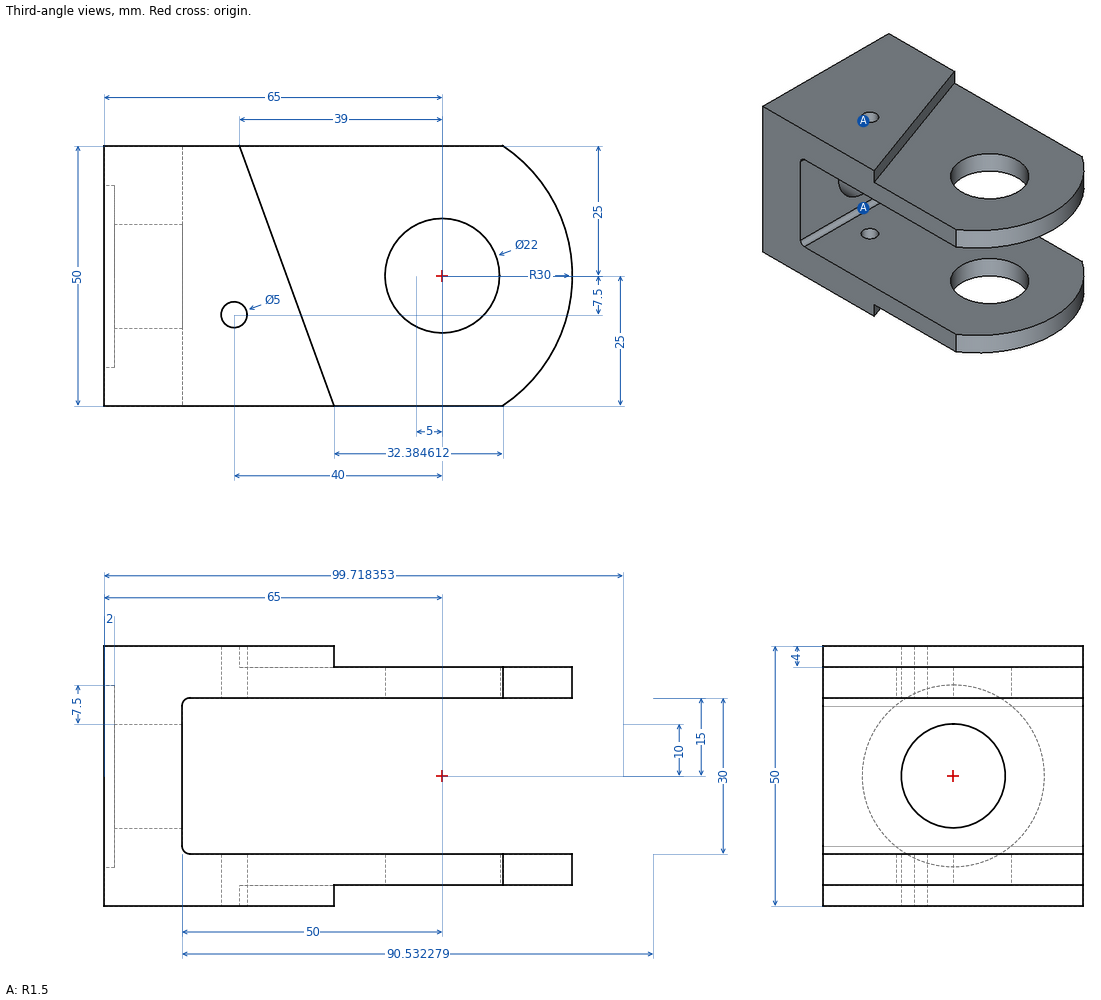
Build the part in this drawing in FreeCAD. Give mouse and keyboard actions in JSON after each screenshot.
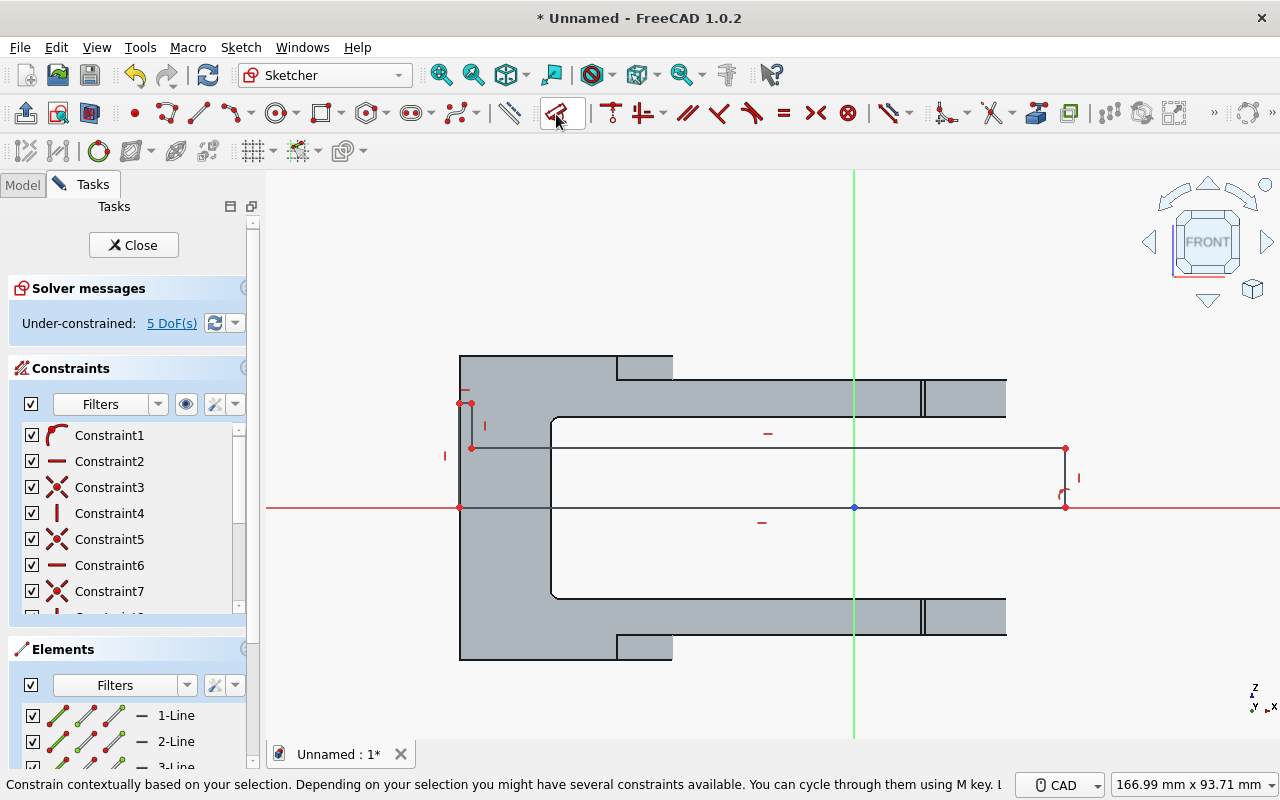
{"action": "scroll", "coordinate": [465, 403], "scroll_direction": "up", "scroll_amount": 6}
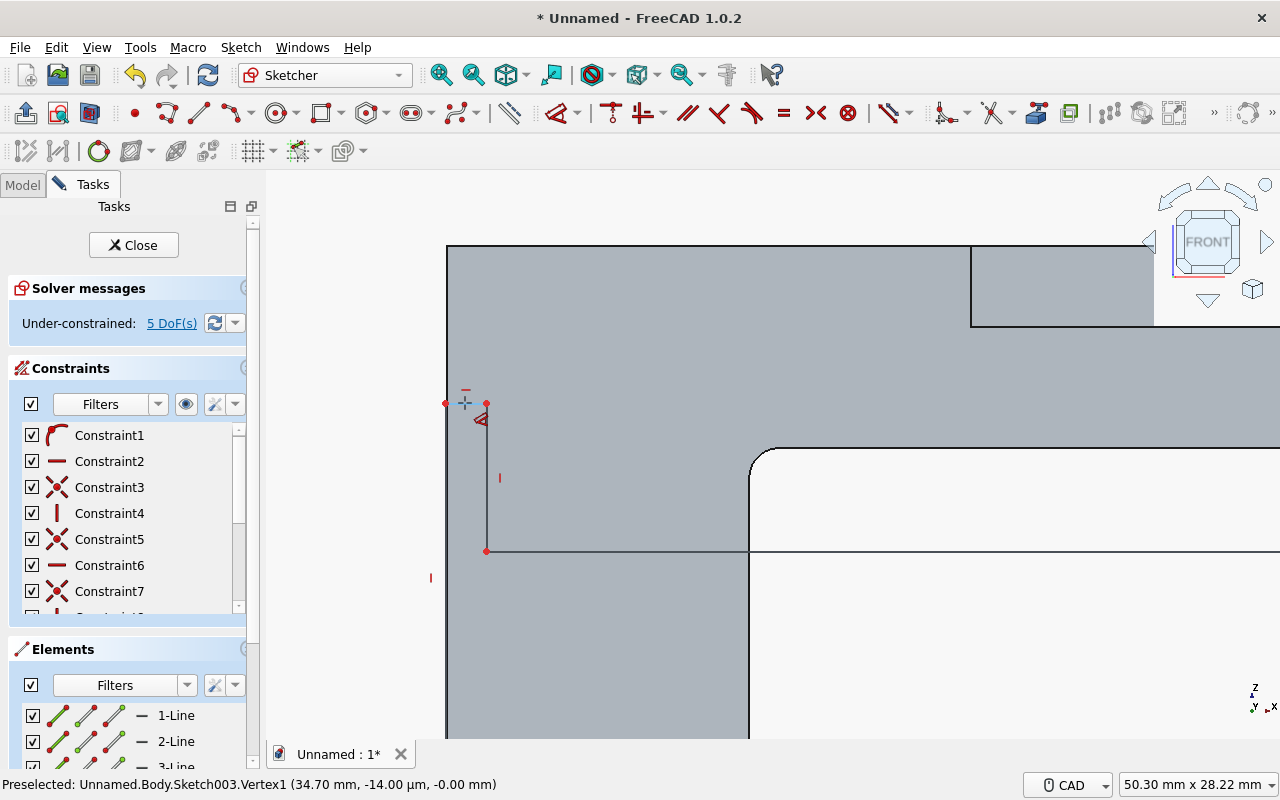
{"action": "left_click", "coordinate": [466, 404]}
{"action": "left_click", "coordinate": [466, 370]}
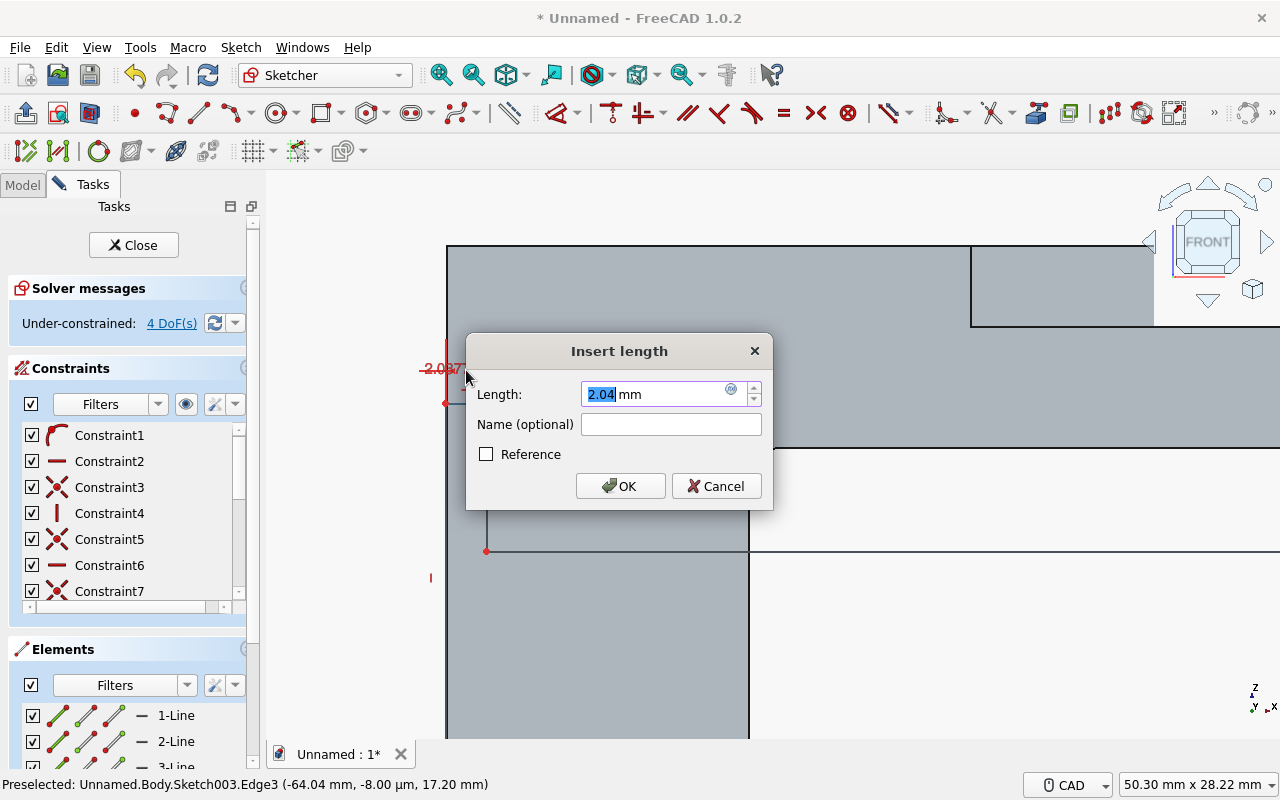
{"action": "type", "text": "2"}
{"action": "key", "text": "Return"}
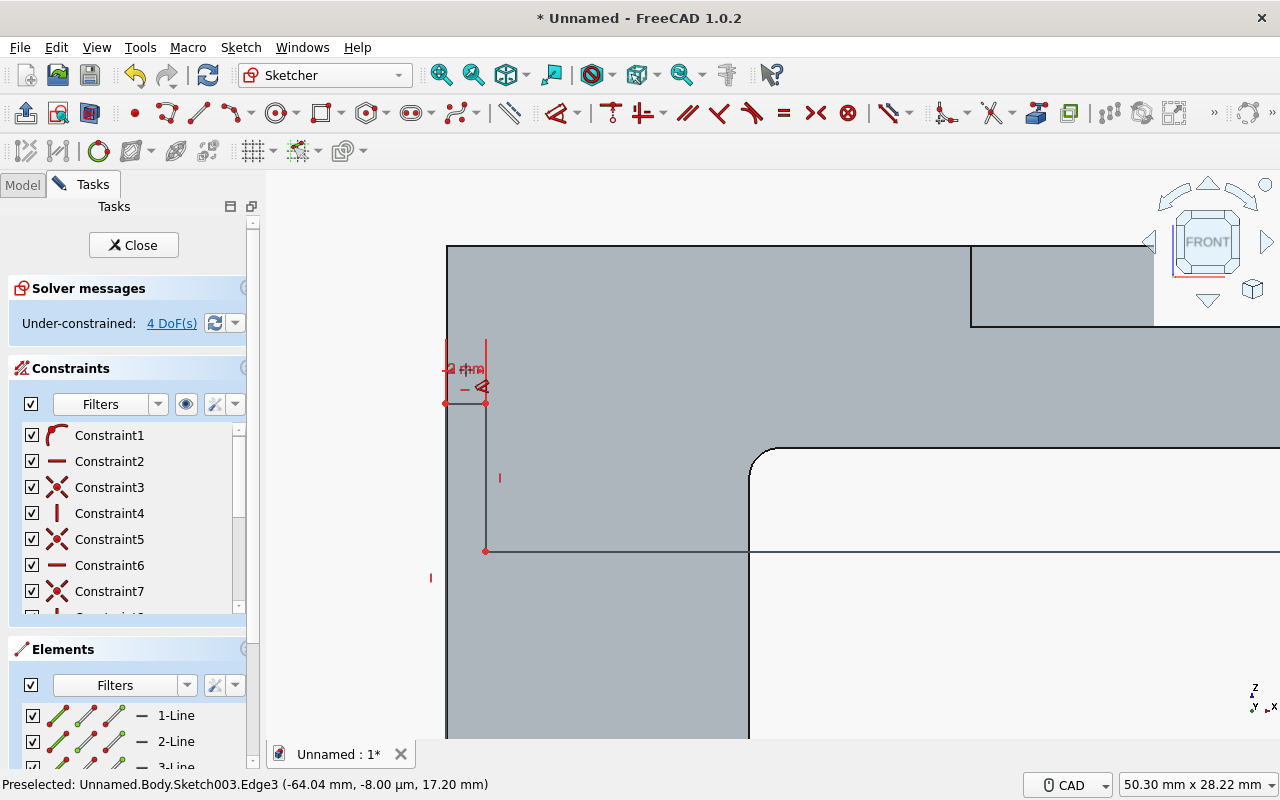
{"action": "scroll", "coordinate": [382, 403], "scroll_direction": "down", "scroll_amount": 6}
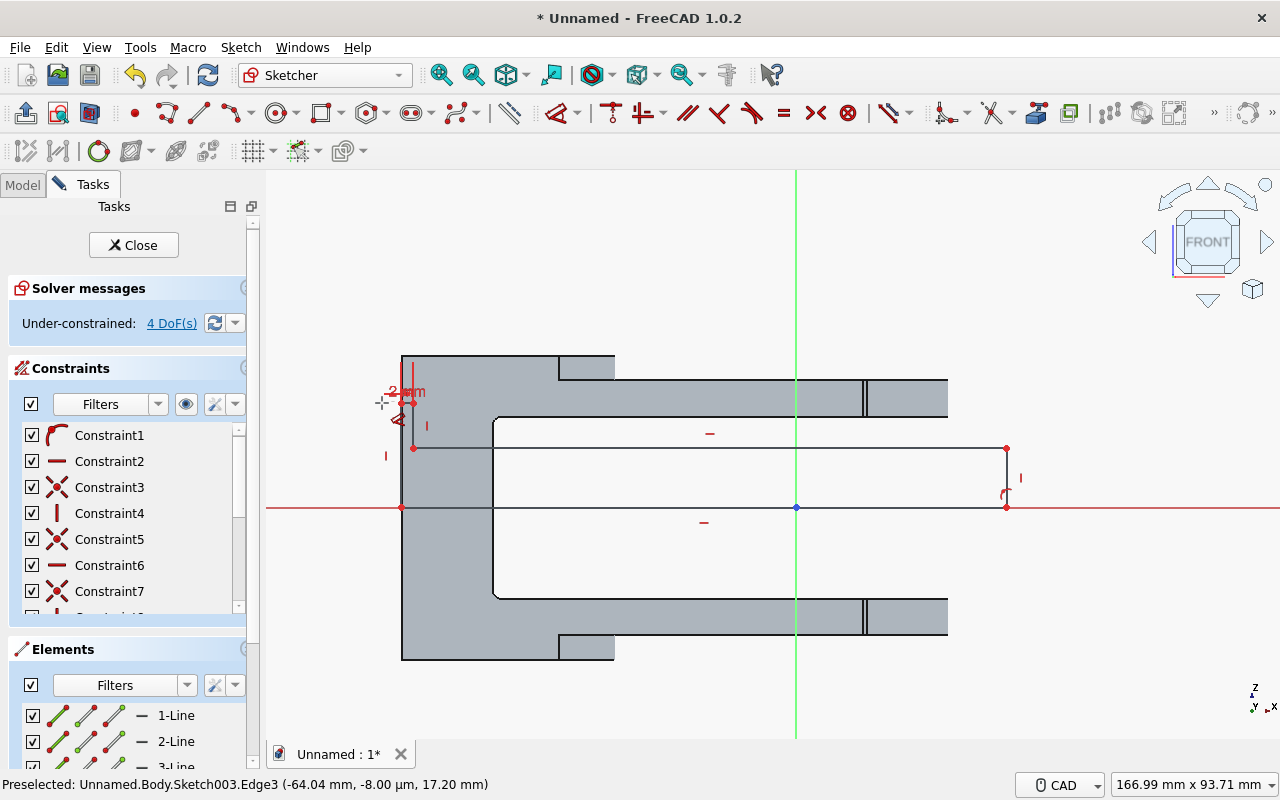
{"action": "left_click", "coordinate": [1007, 466]}
{"action": "left_click", "coordinate": [1041, 478]}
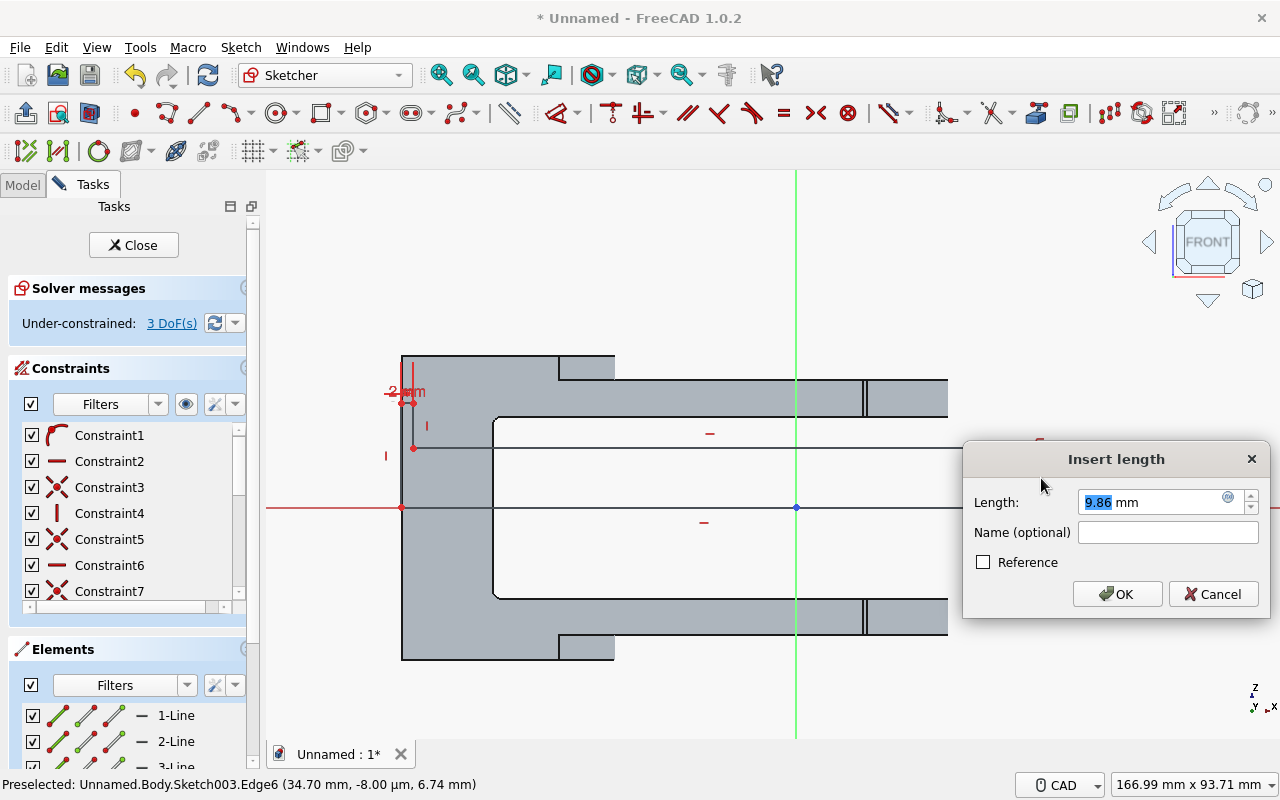
{"action": "type", "text": "10"}
{"action": "key", "text": "Return"}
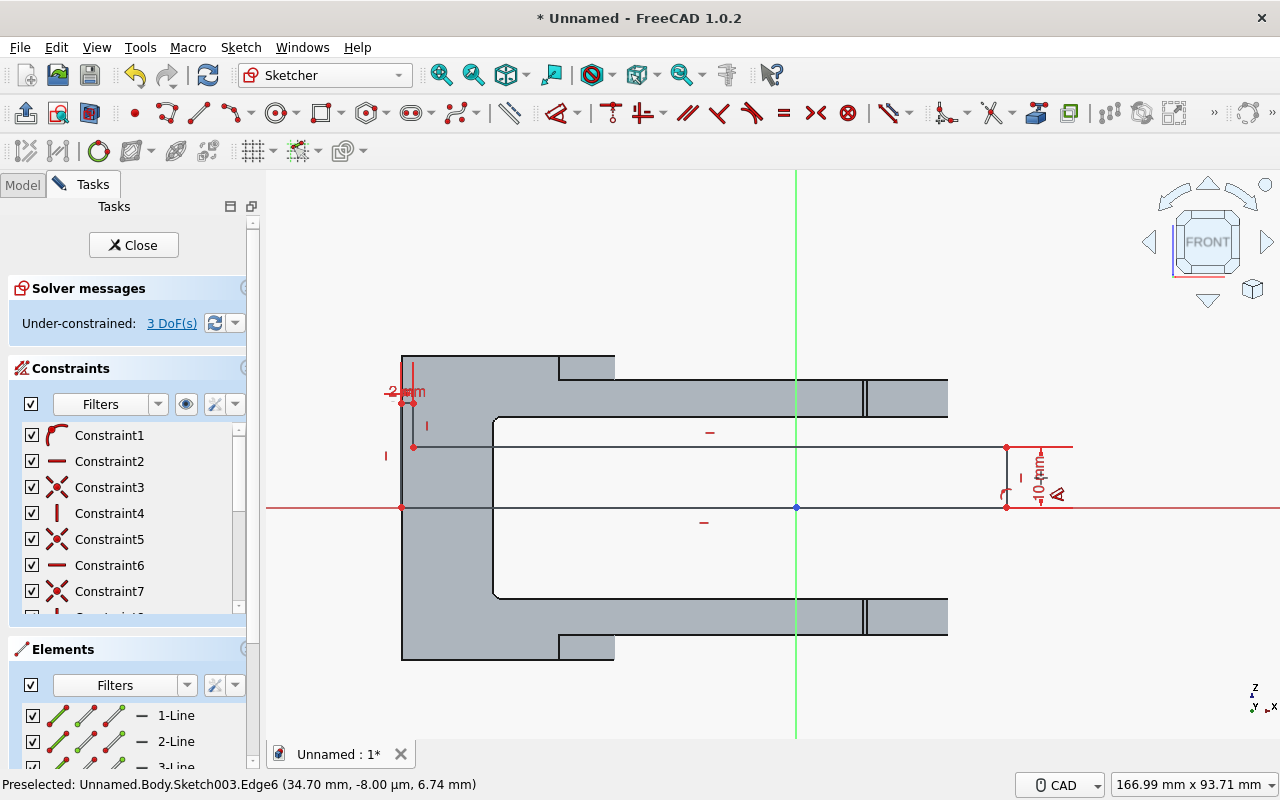
{"action": "left_click", "coordinate": [413, 417]}
{"action": "left_click", "coordinate": [379, 425]}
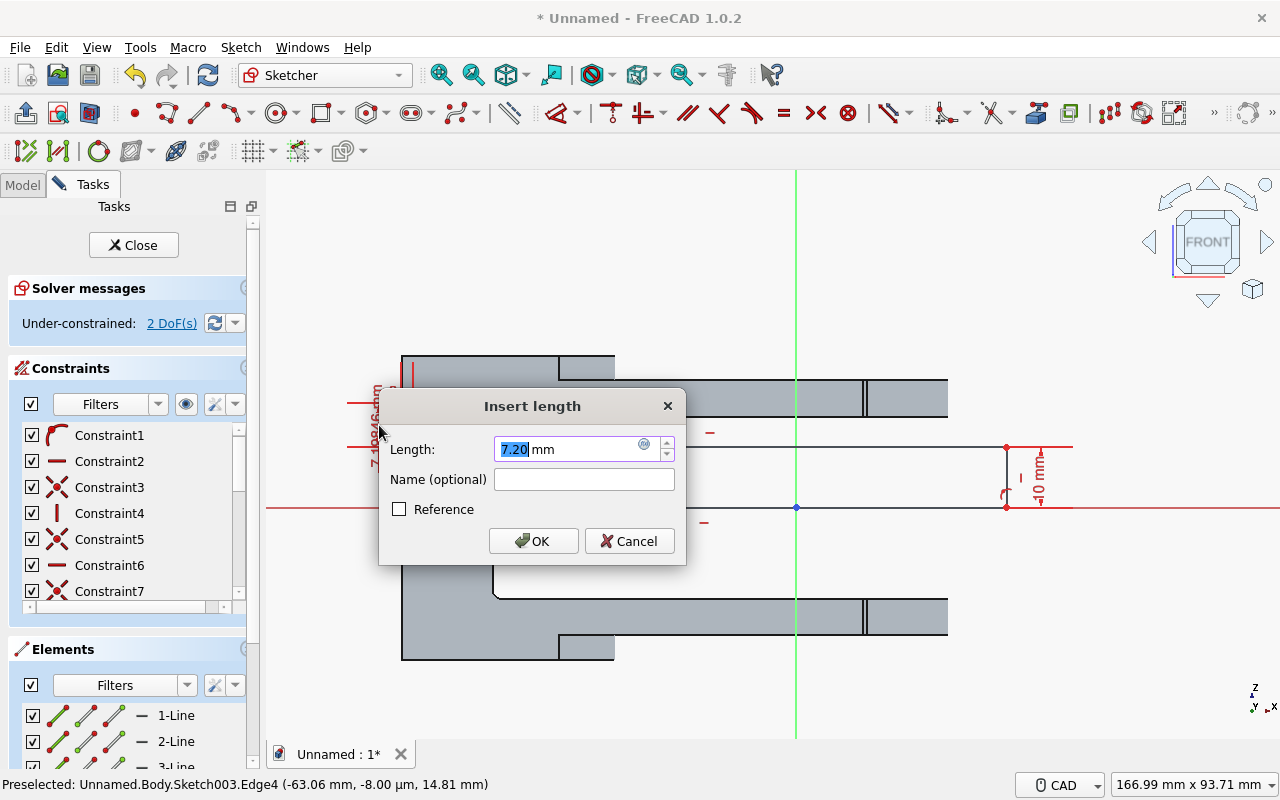
{"action": "type", "text": "7.5"}
{"action": "key", "text": "Return"}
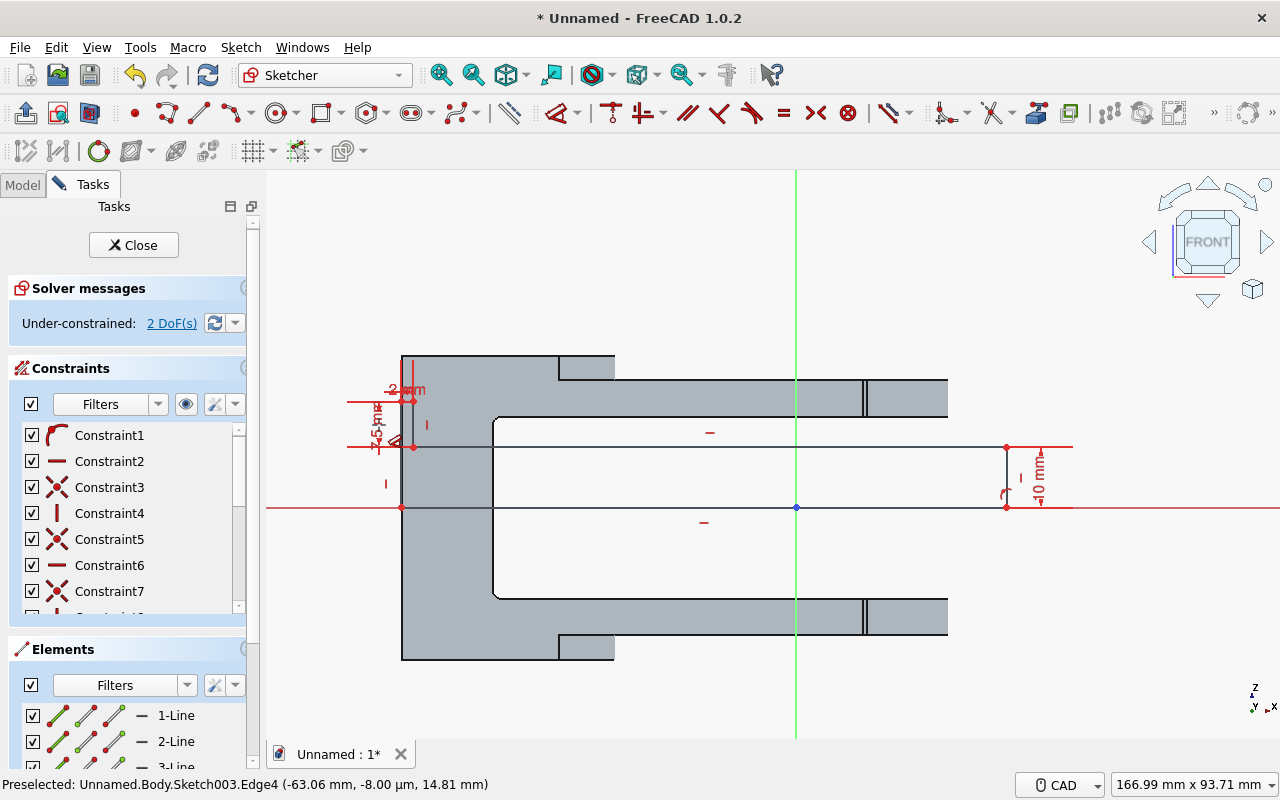
{"action": "left_click", "coordinate": [401, 508]}
{"action": "left_click", "coordinate": [599, 542]}